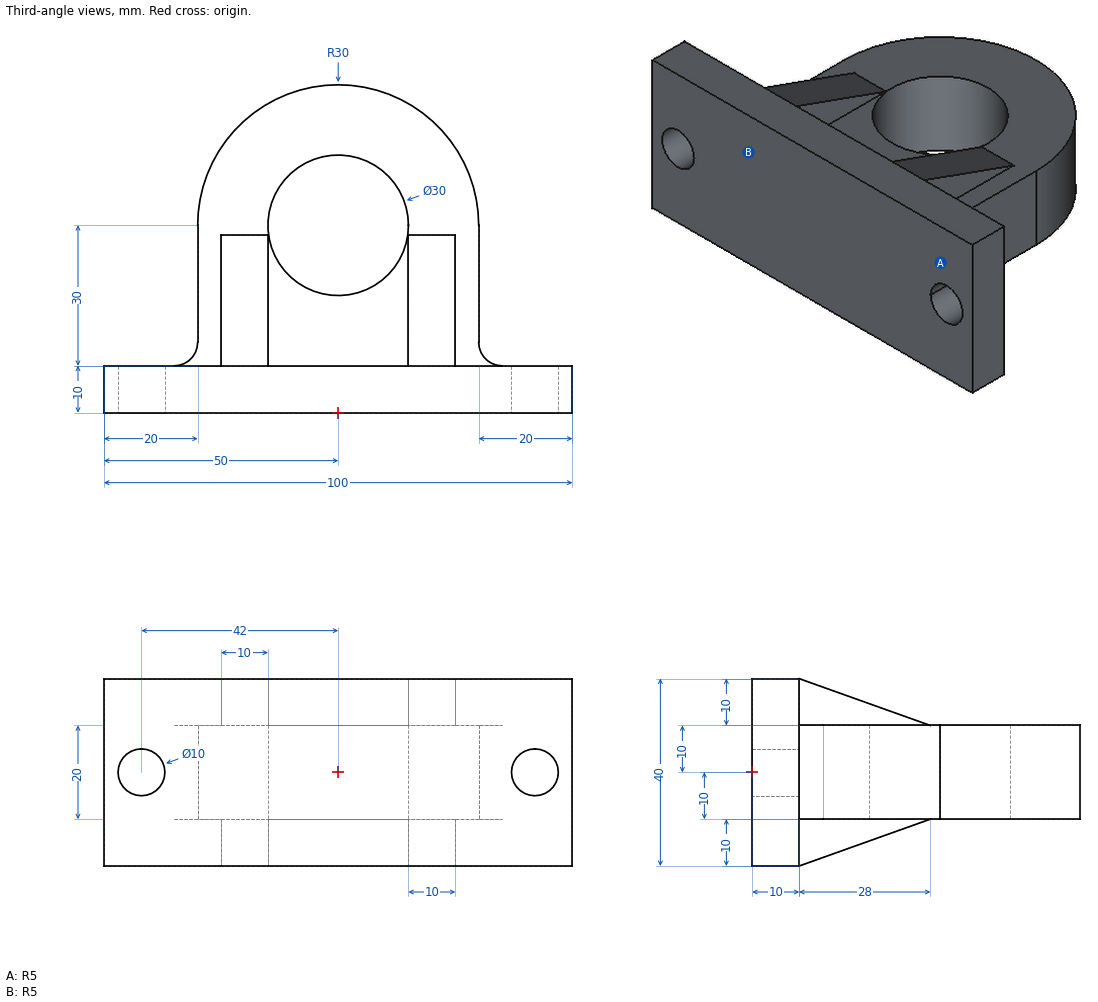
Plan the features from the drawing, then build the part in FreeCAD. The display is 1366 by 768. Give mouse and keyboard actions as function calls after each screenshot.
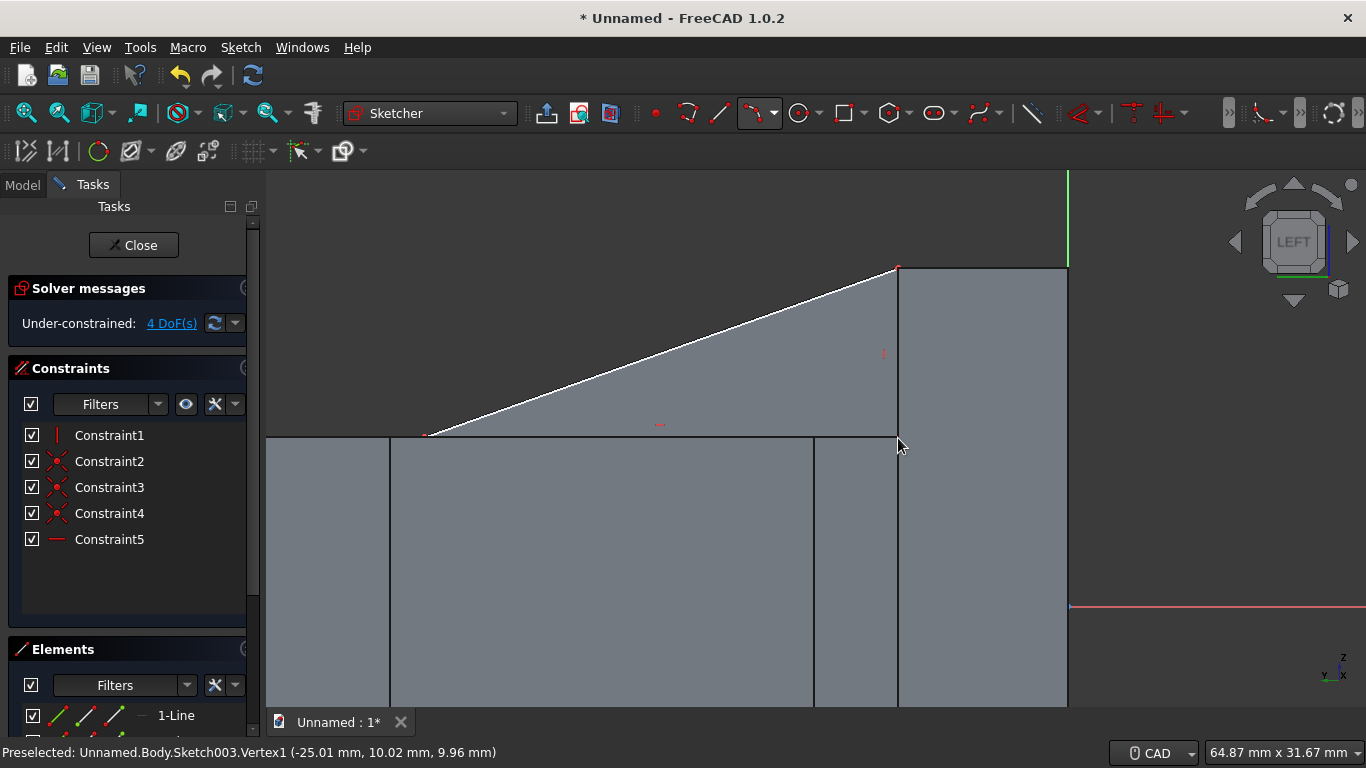
click(1078, 114)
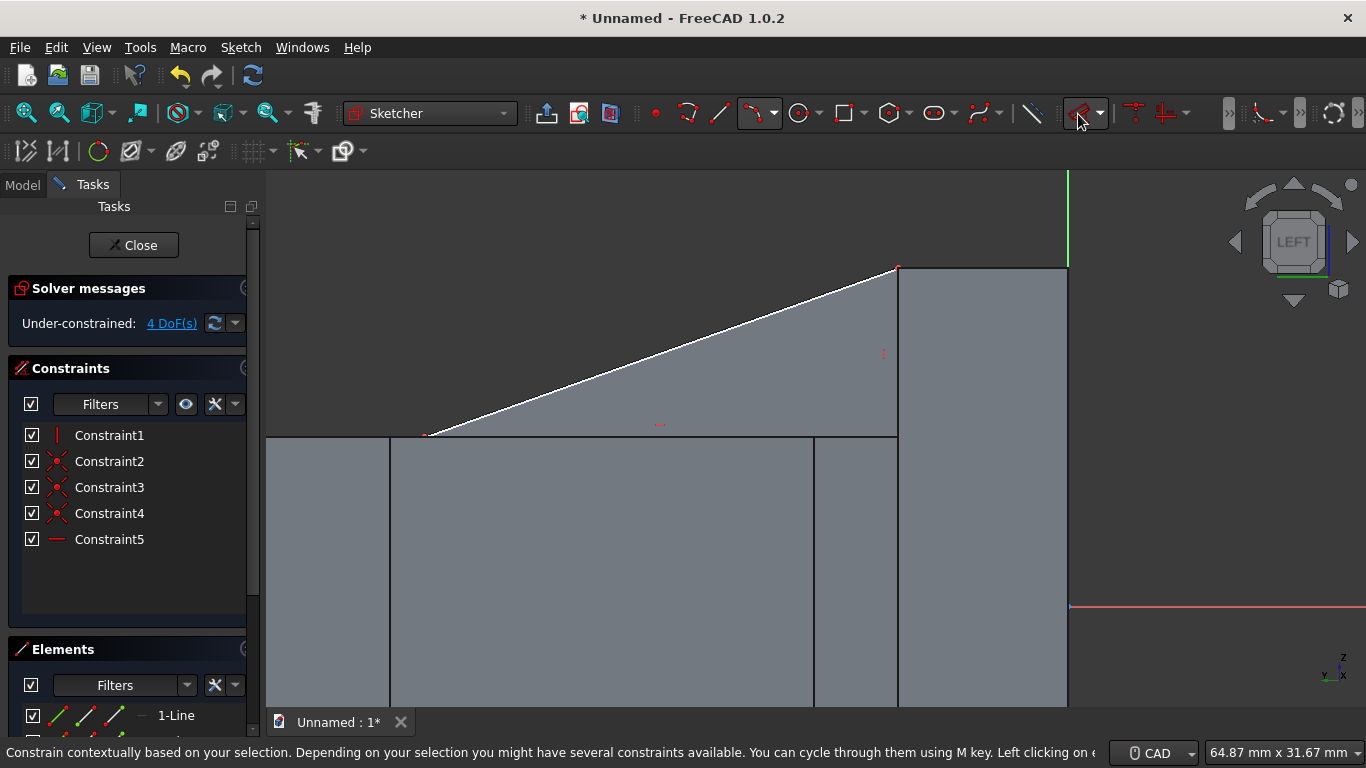
click(898, 387)
click(932, 354)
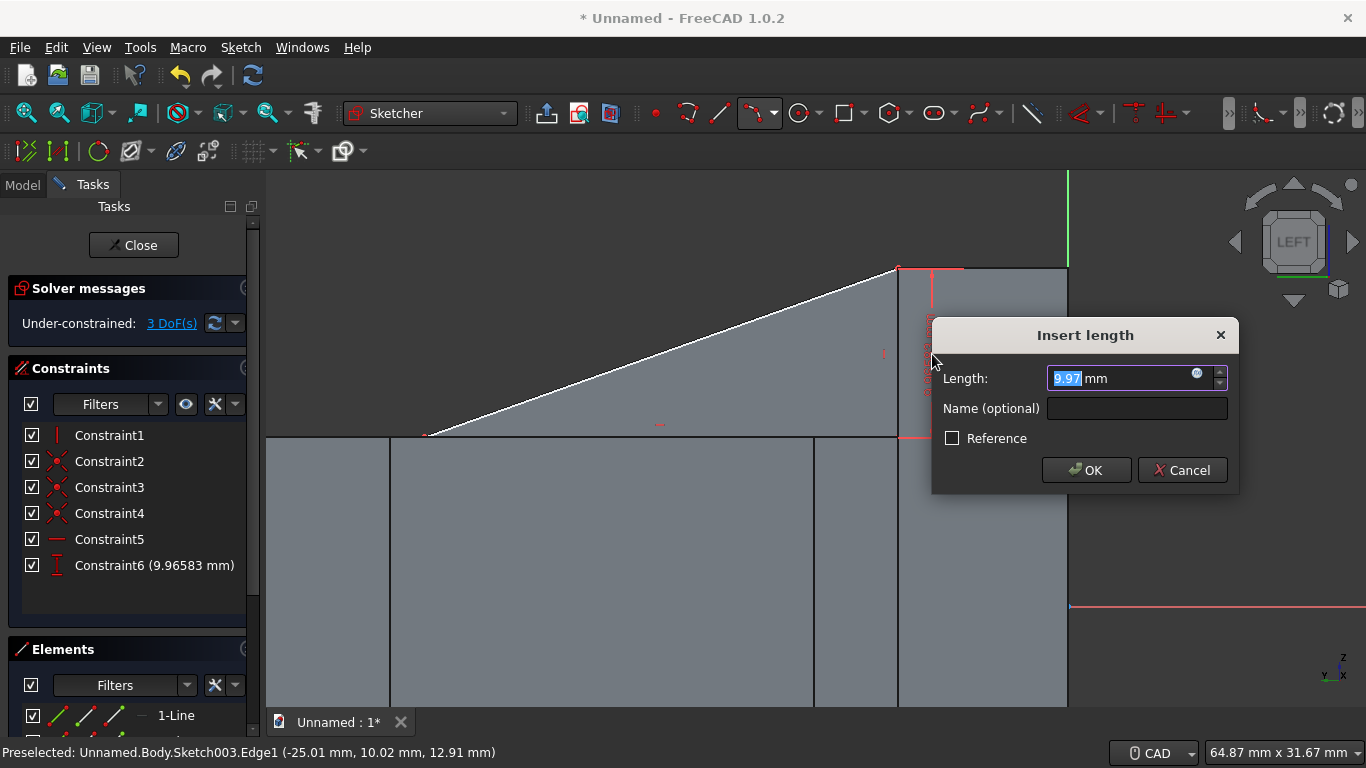
text(10)
key(Return)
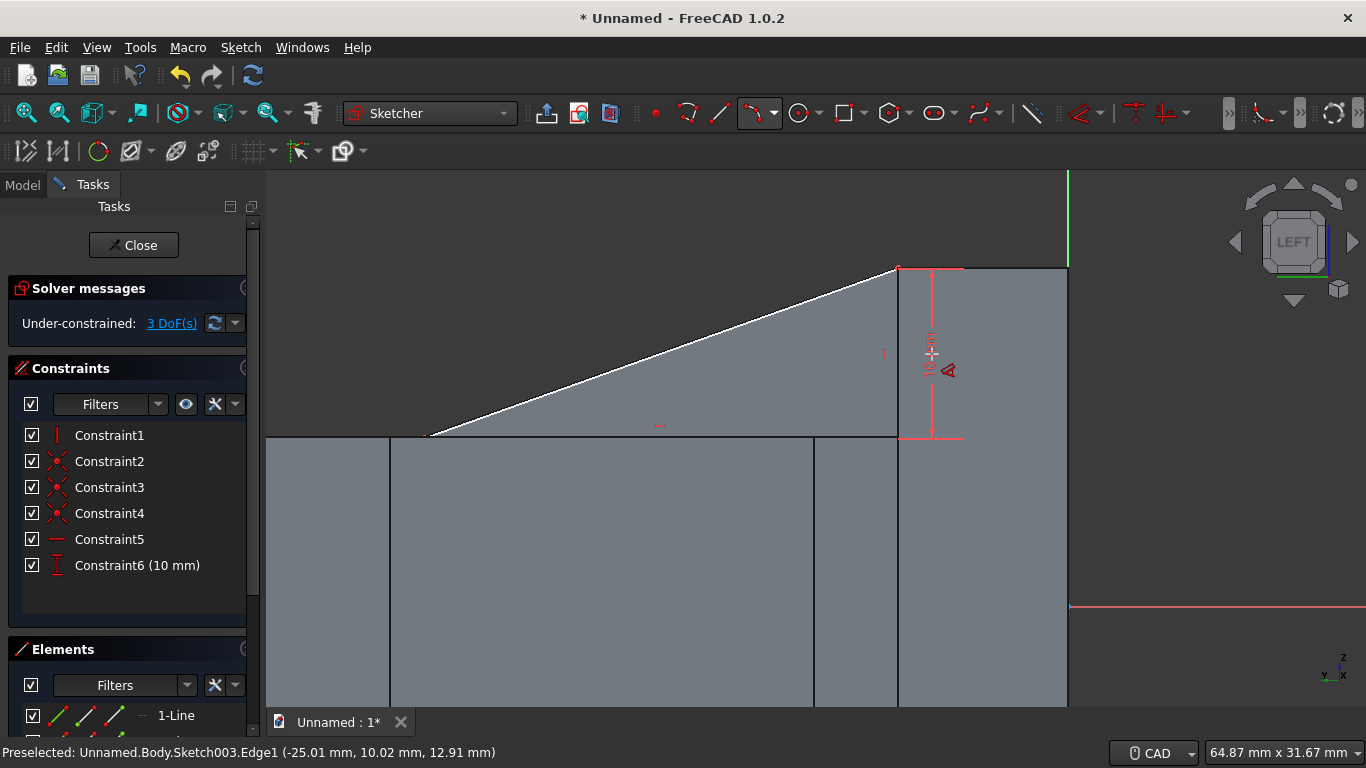
click(566, 439)
click(661, 473)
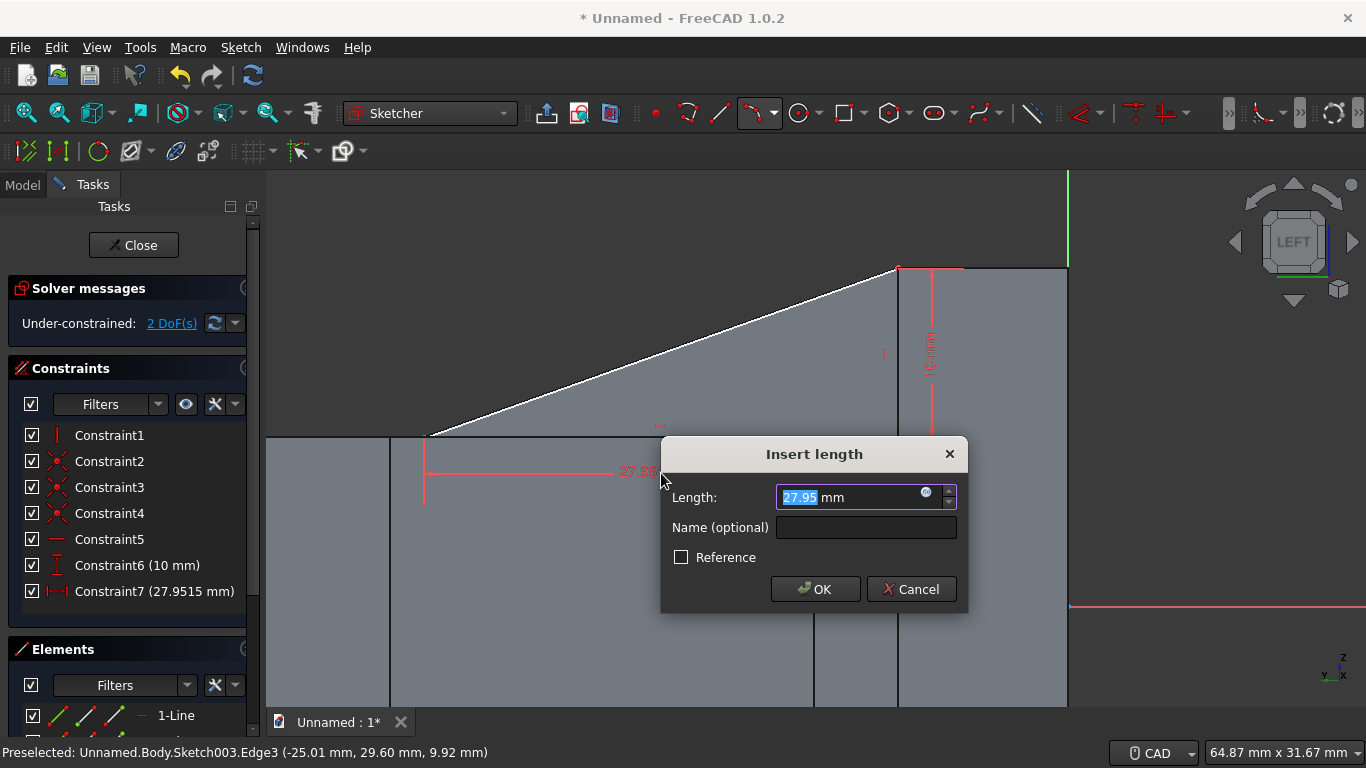
text(28)
key(Return)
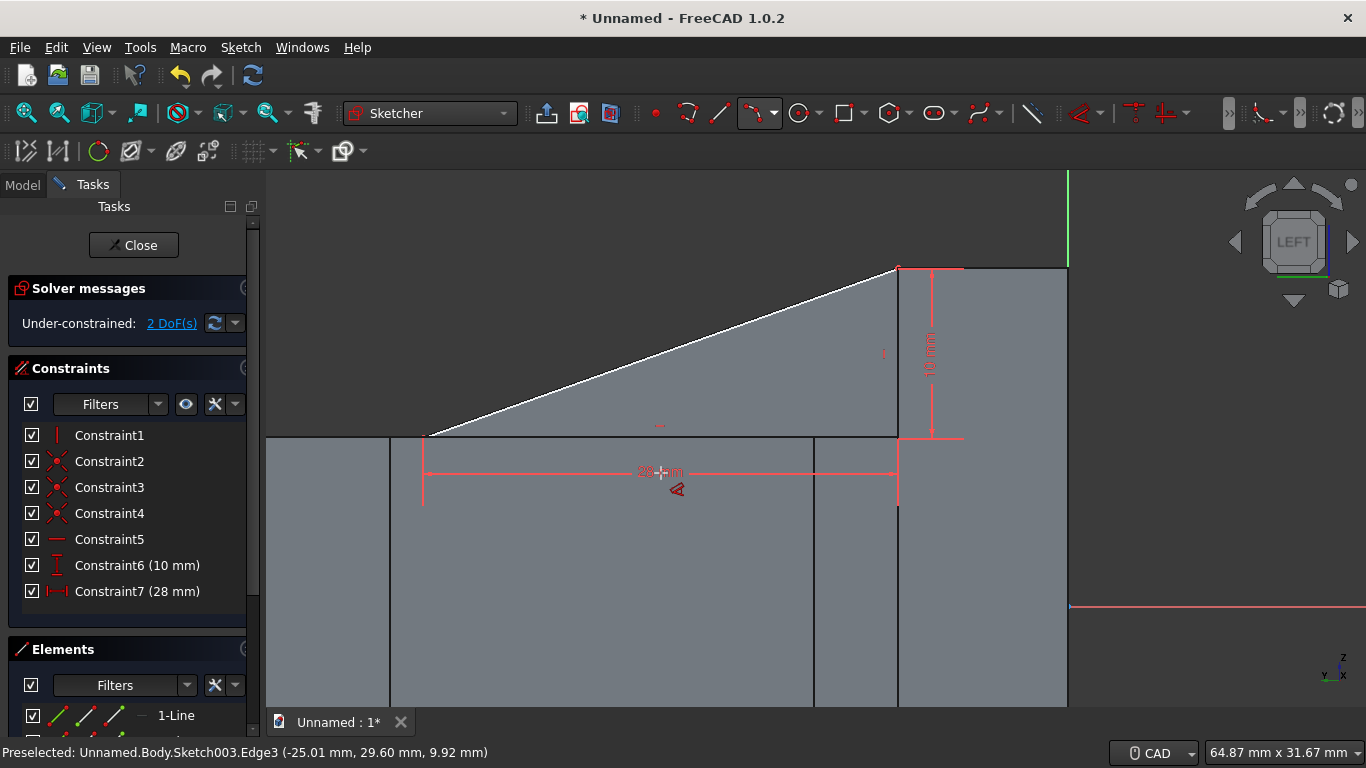
click(898, 439)
click(983, 641)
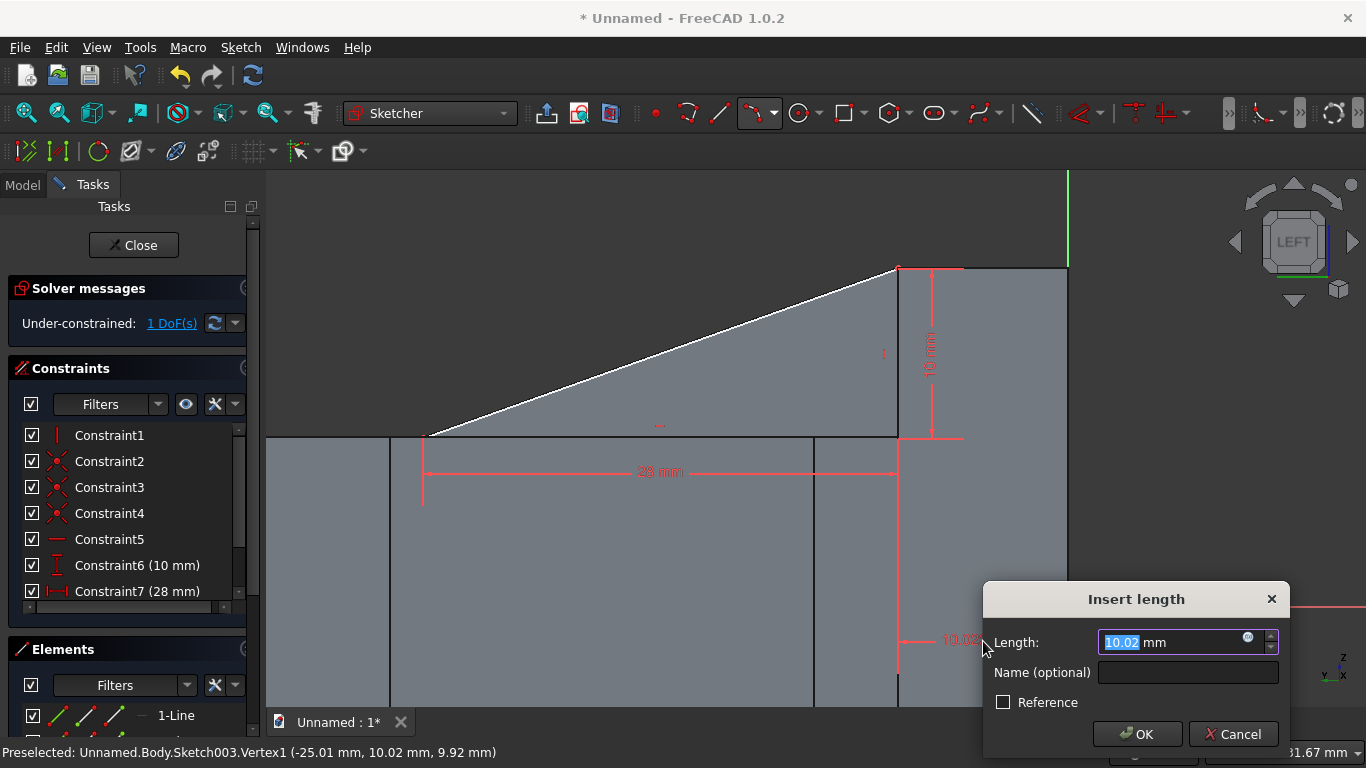
text(10)
key(Return)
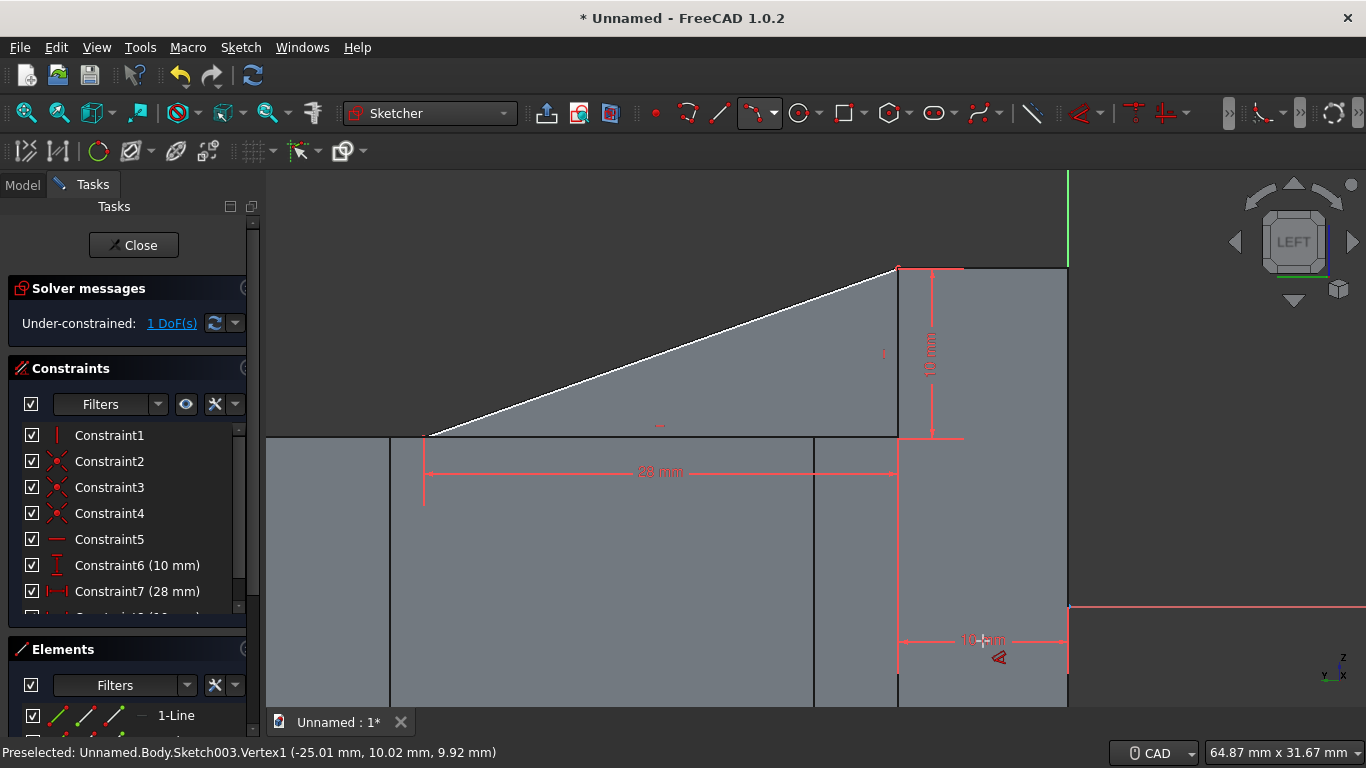
click(898, 439)
click(1102, 523)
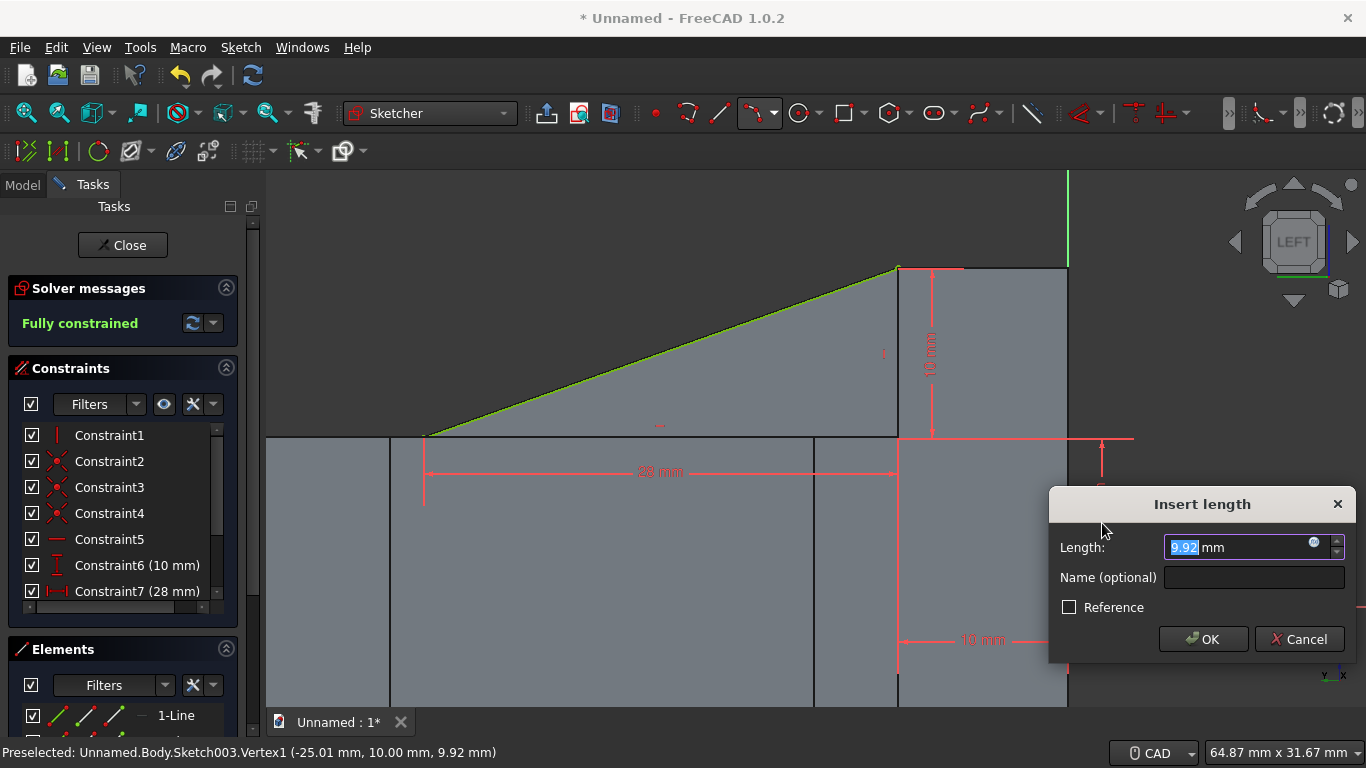
text(10)
key(Return)
key(Escape)